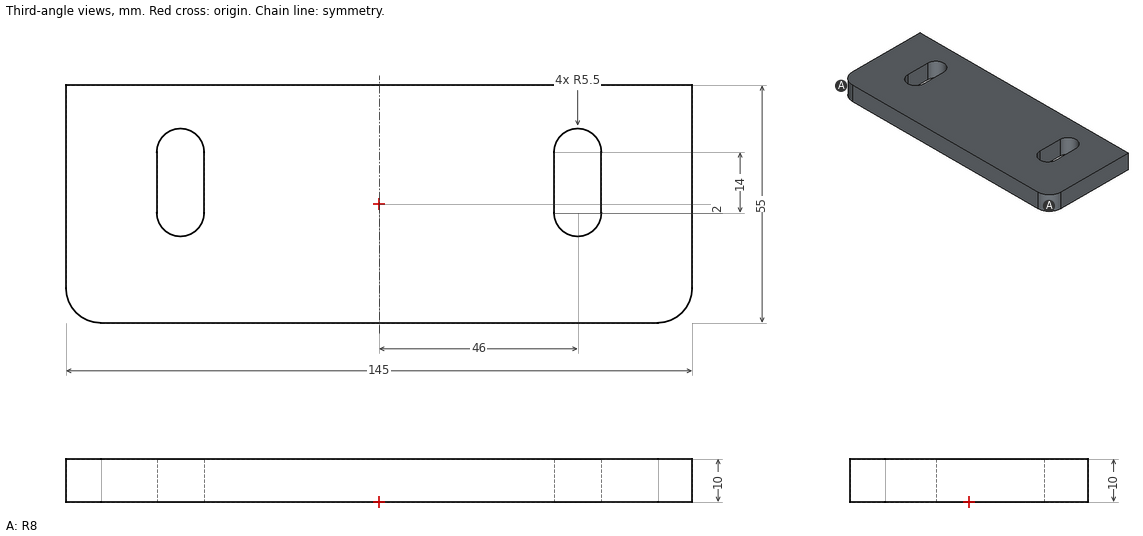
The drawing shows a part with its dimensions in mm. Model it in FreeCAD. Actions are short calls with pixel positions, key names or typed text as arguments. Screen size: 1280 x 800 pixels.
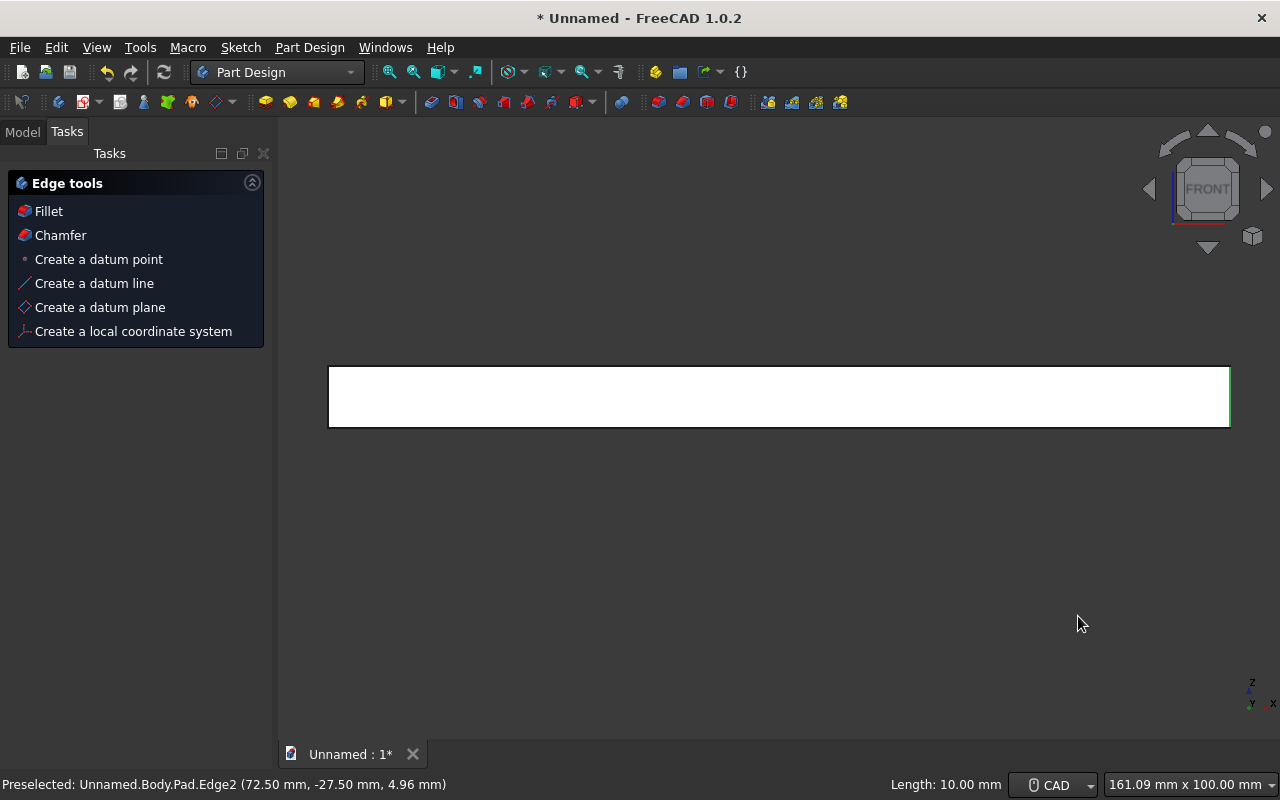
click(328, 396, ctrl)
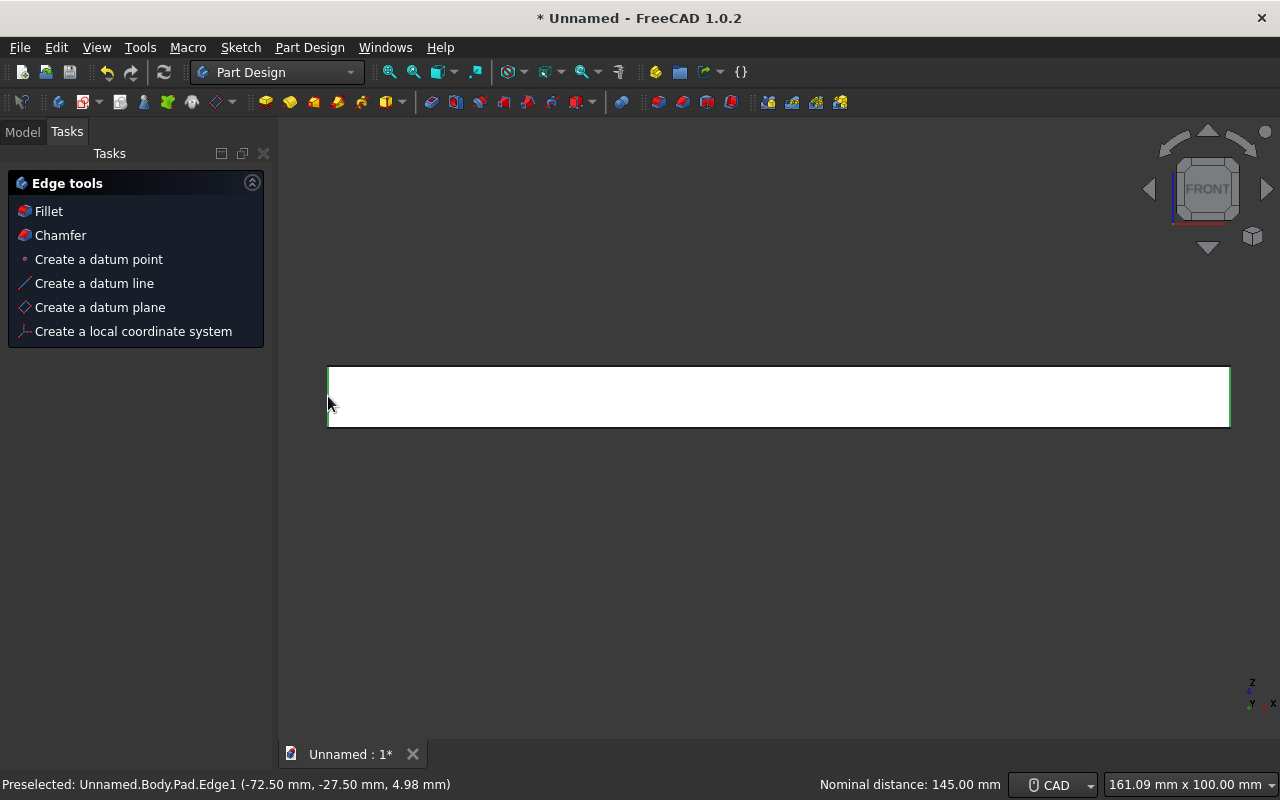
click(660, 102)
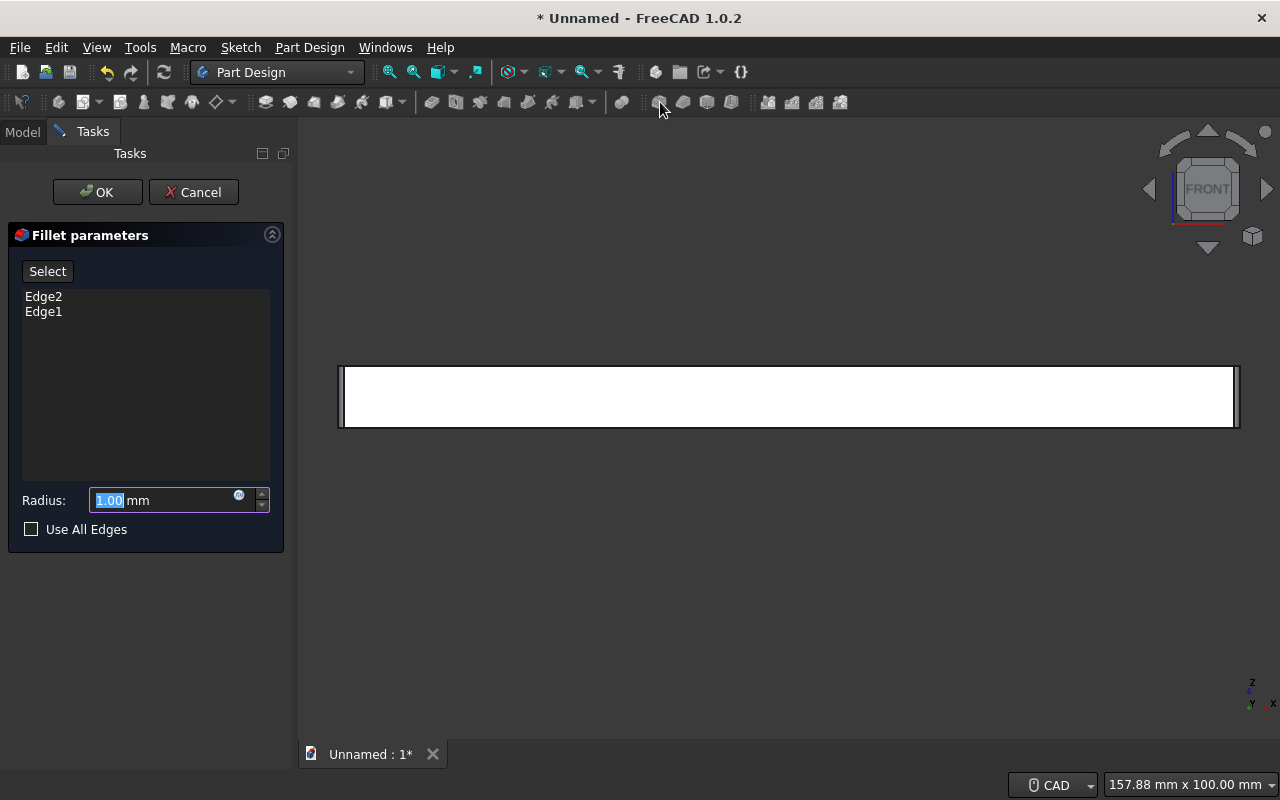
text(8)
key(Tab)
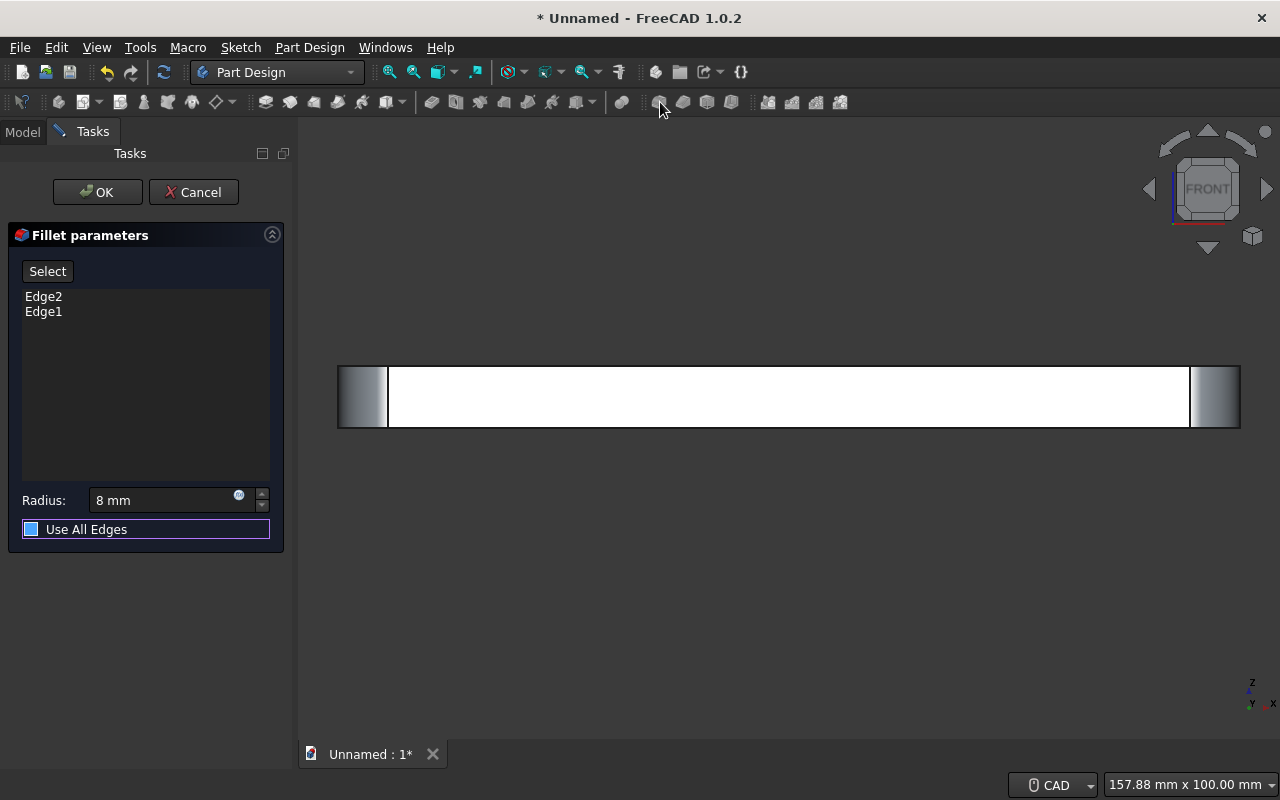
click(98, 192)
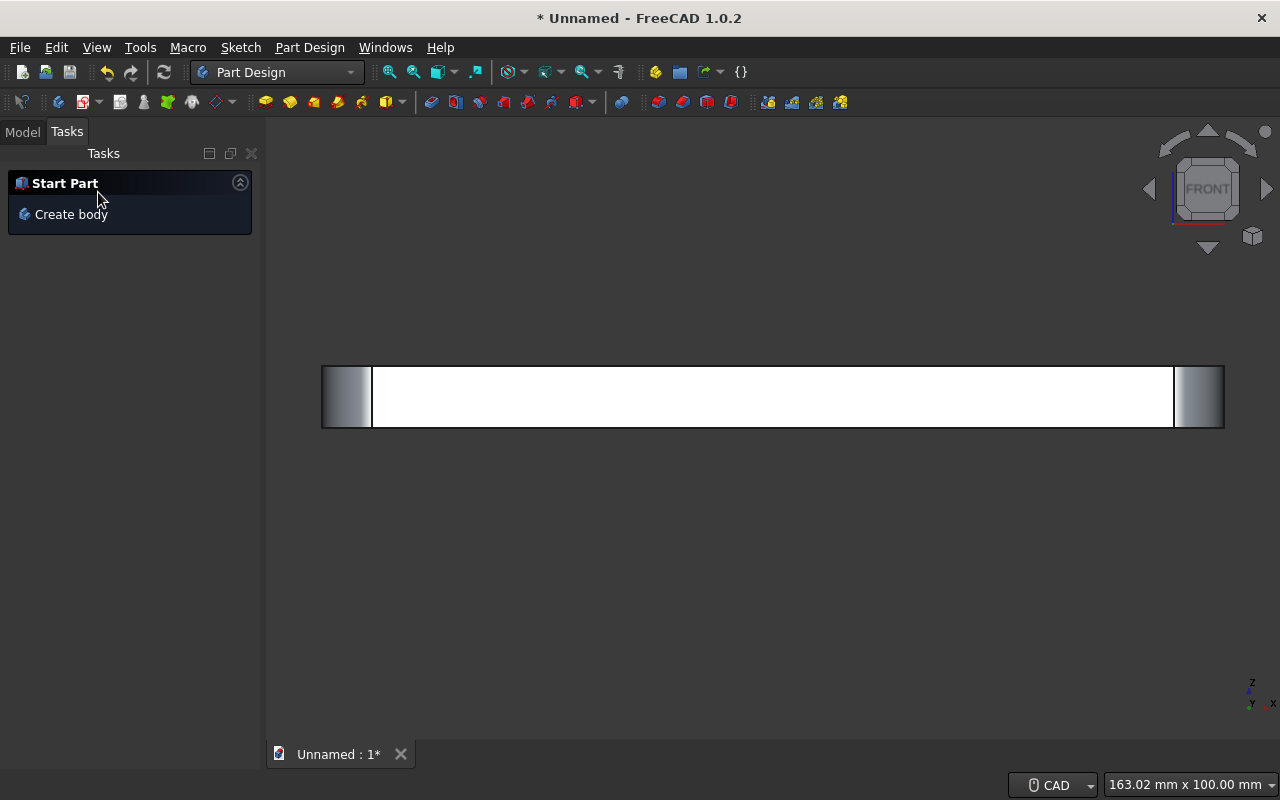
key(0)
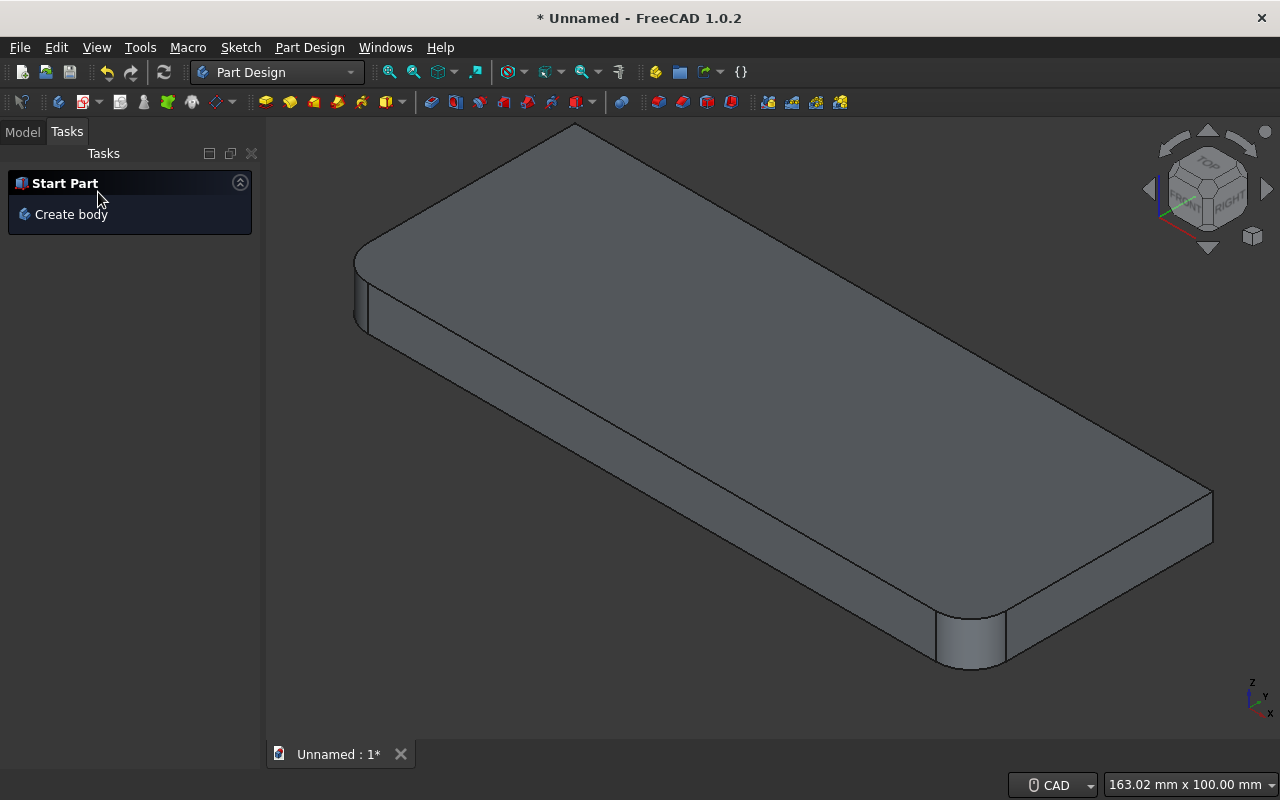
click(955, 481)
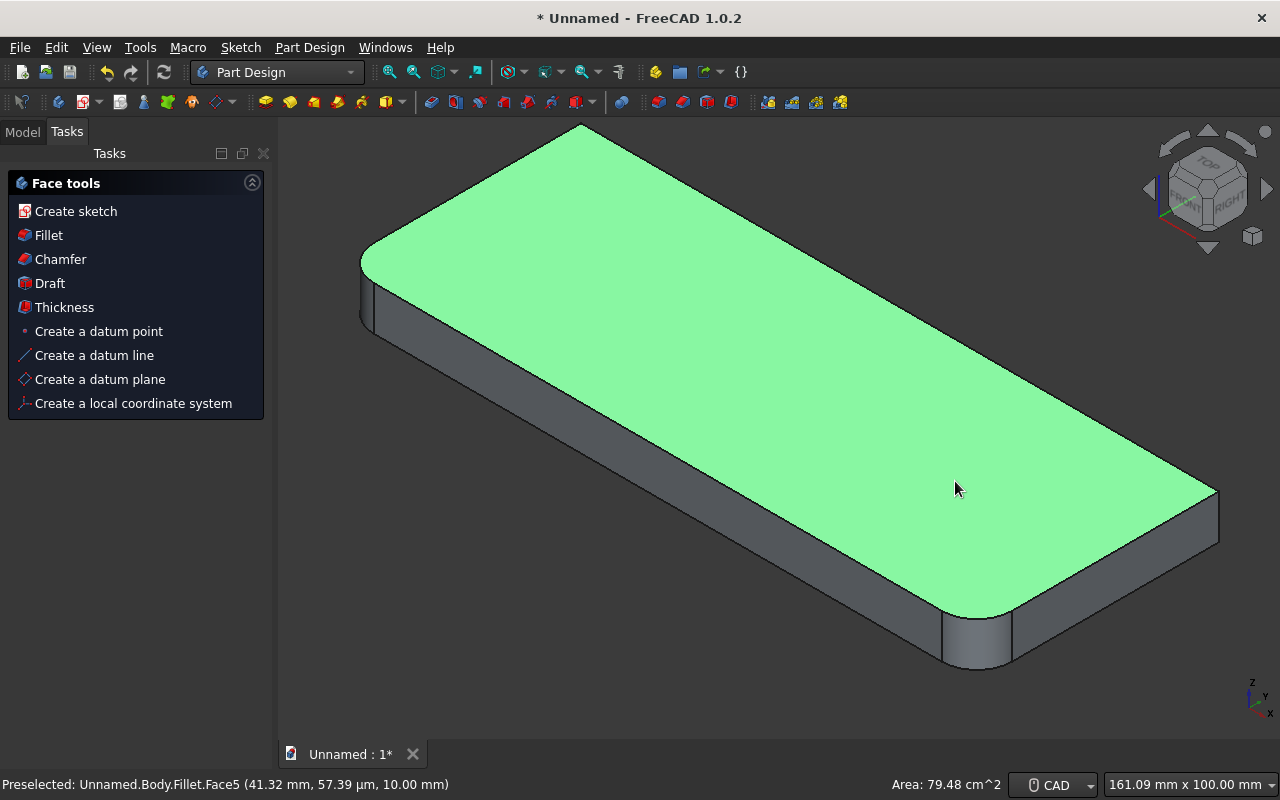
click(84, 102)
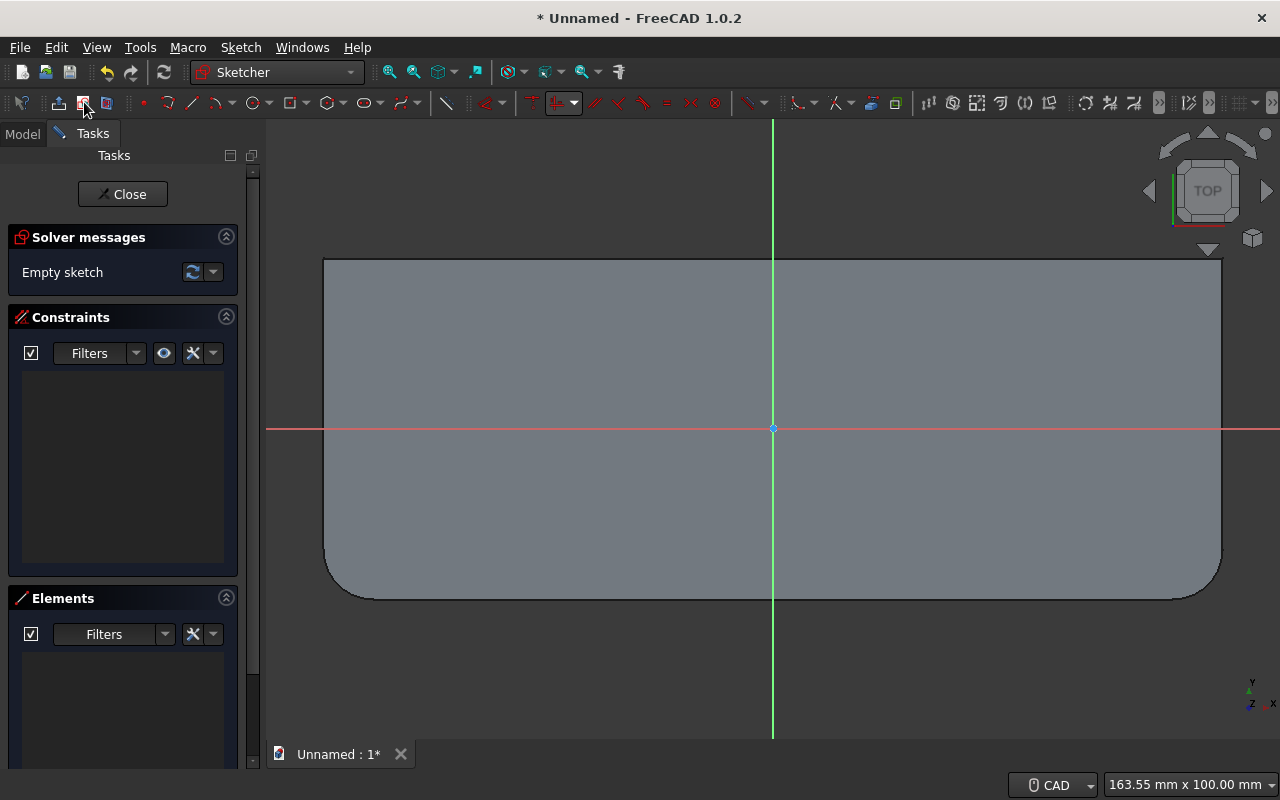
scroll(395, 569, down, 1)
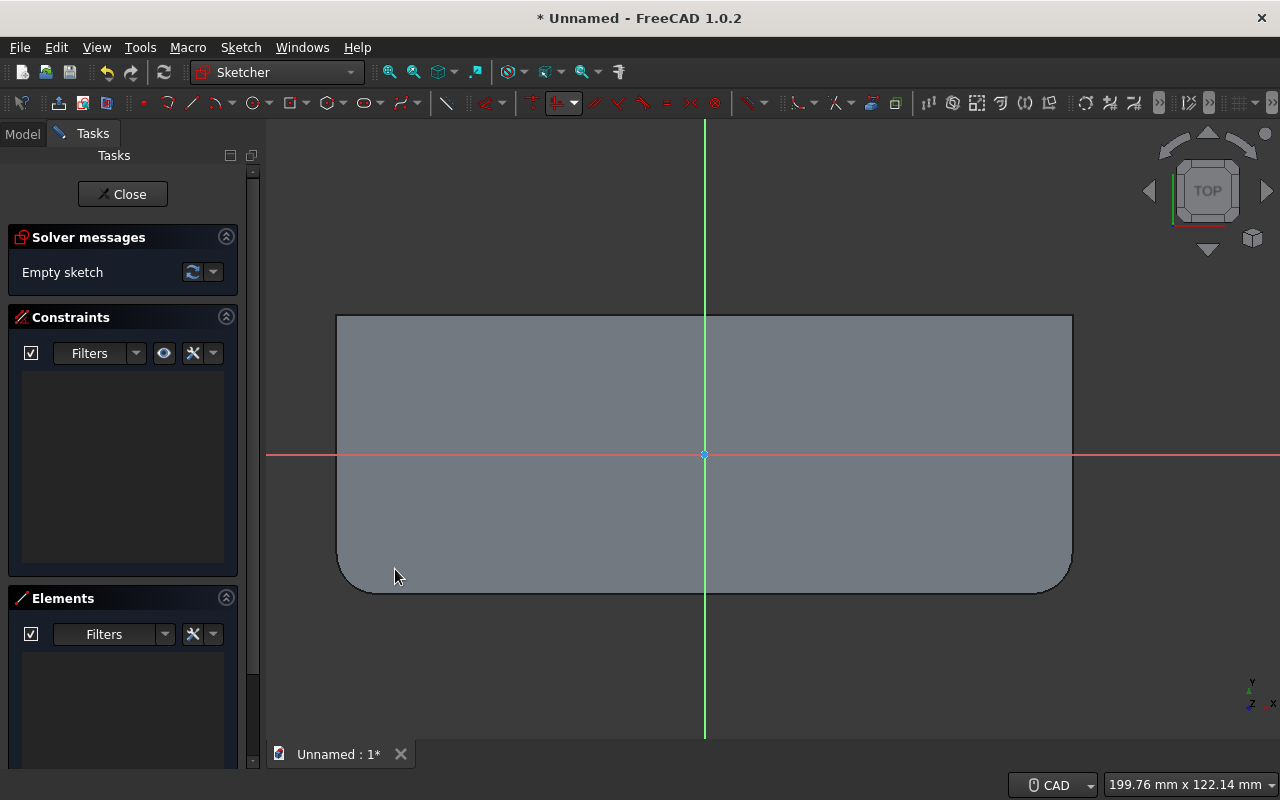
click(364, 104)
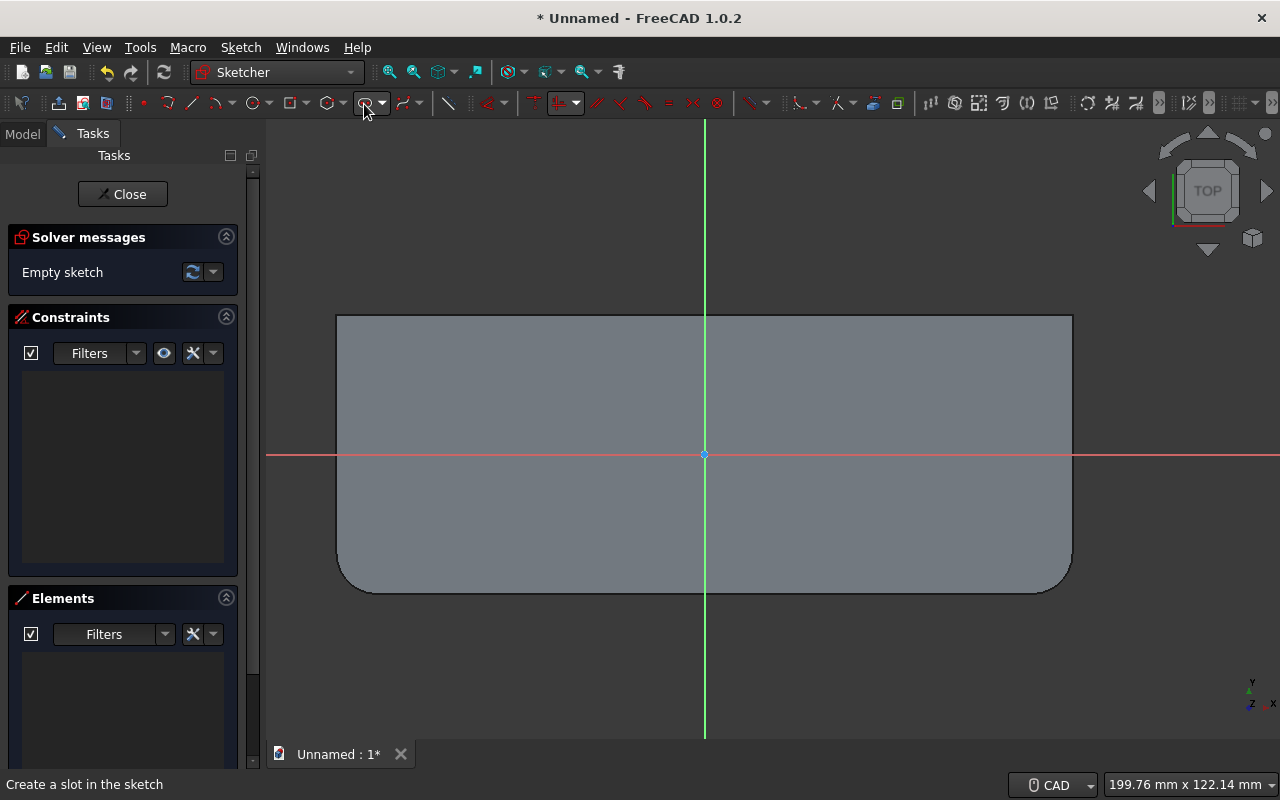
scroll(938, 465, up, 3)